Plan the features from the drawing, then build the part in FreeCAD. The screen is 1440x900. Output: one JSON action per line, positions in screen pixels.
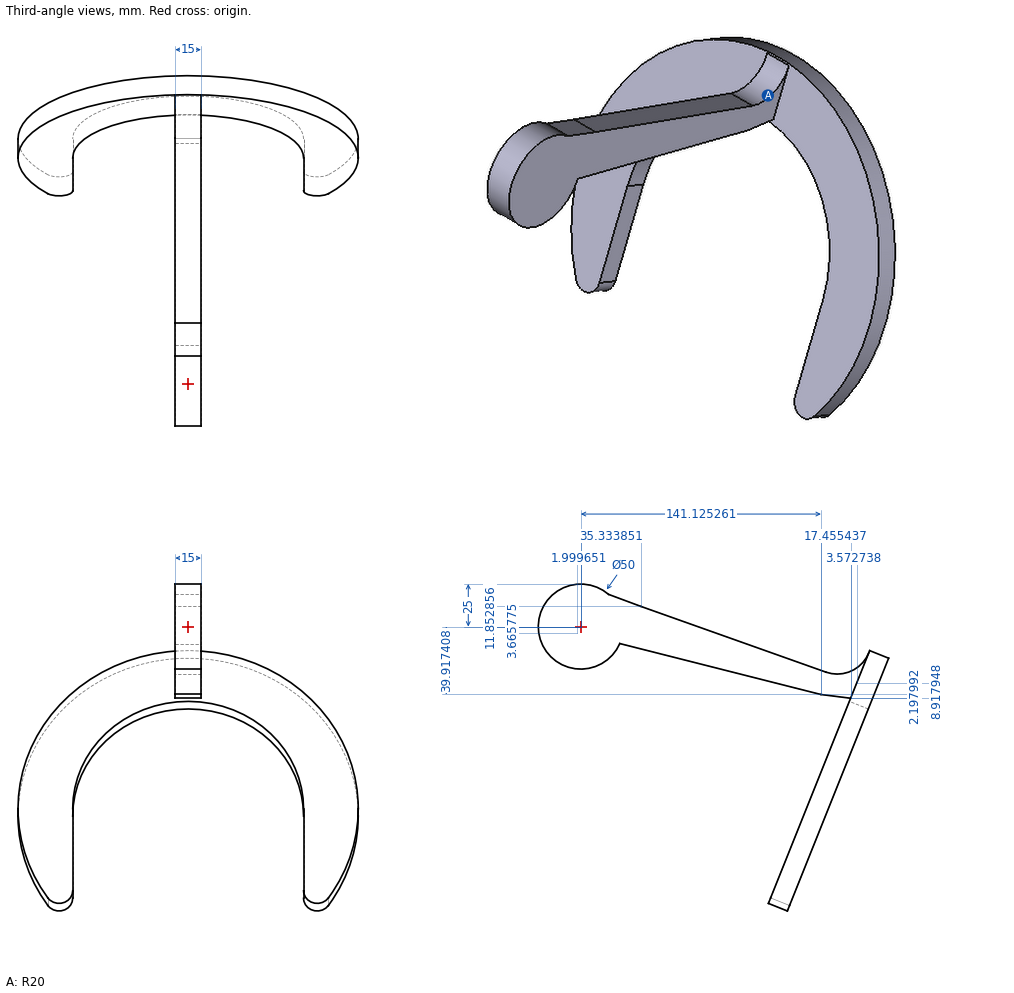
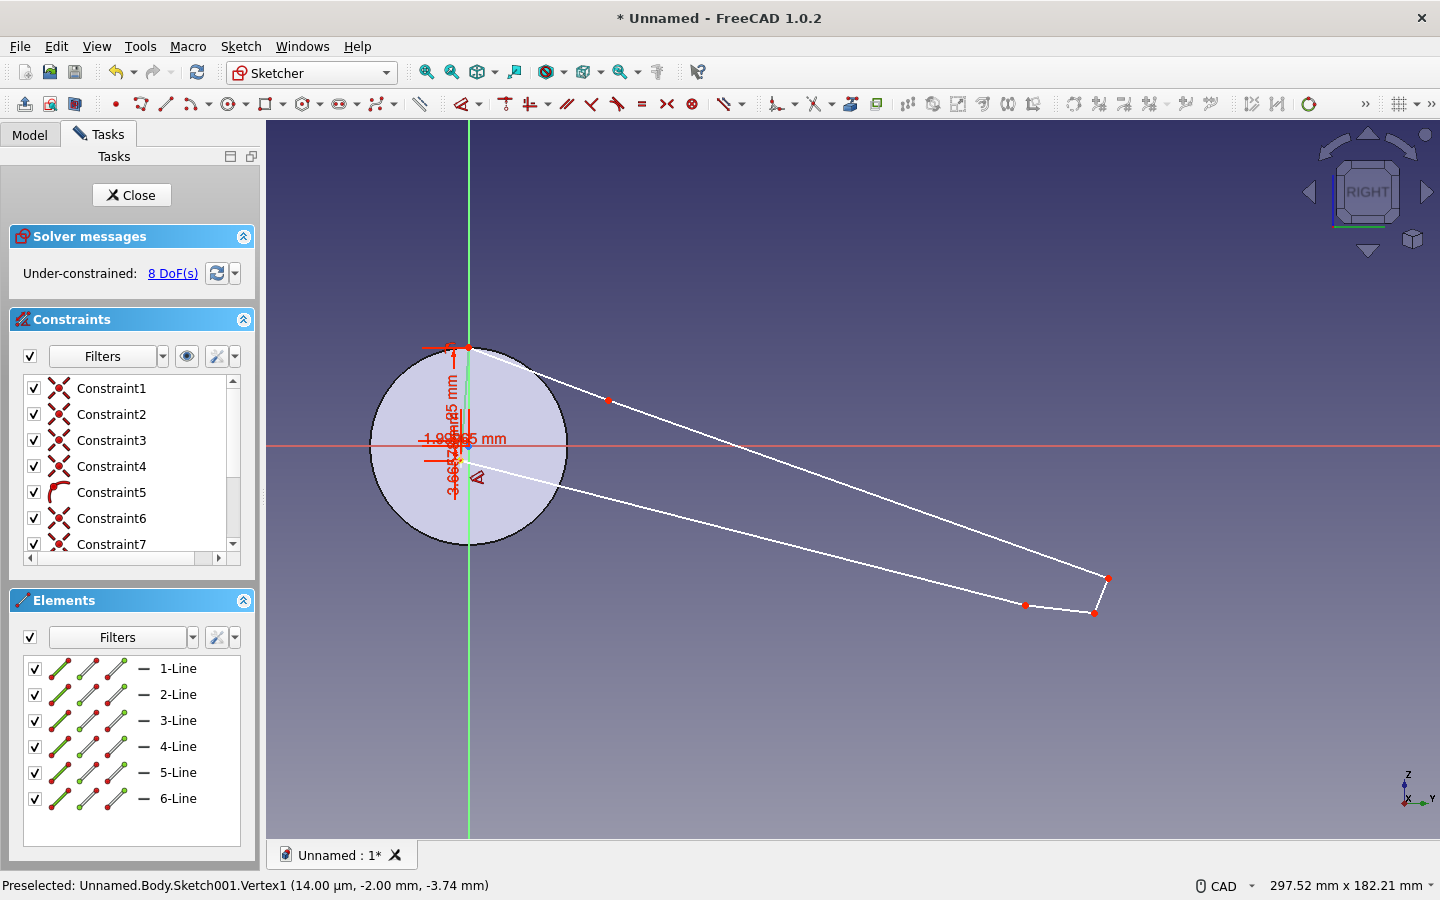
{"action": "scroll", "coordinate": [1046, 608], "scroll_direction": "up", "scroll_amount": 8}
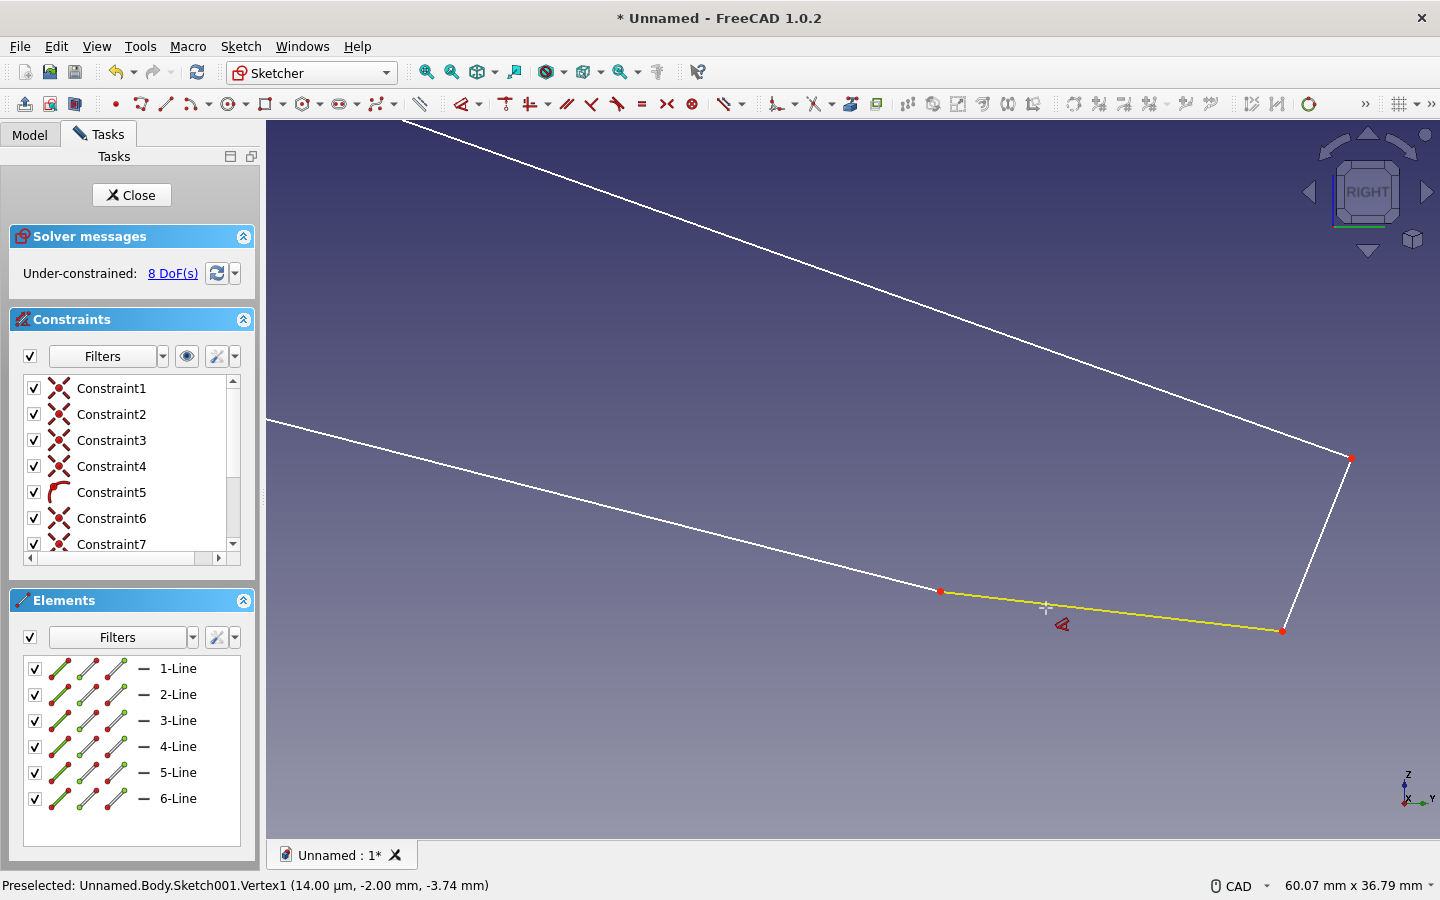
{"action": "left_click", "coordinate": [1043, 604]}
{"action": "left_click", "coordinate": [907, 612]}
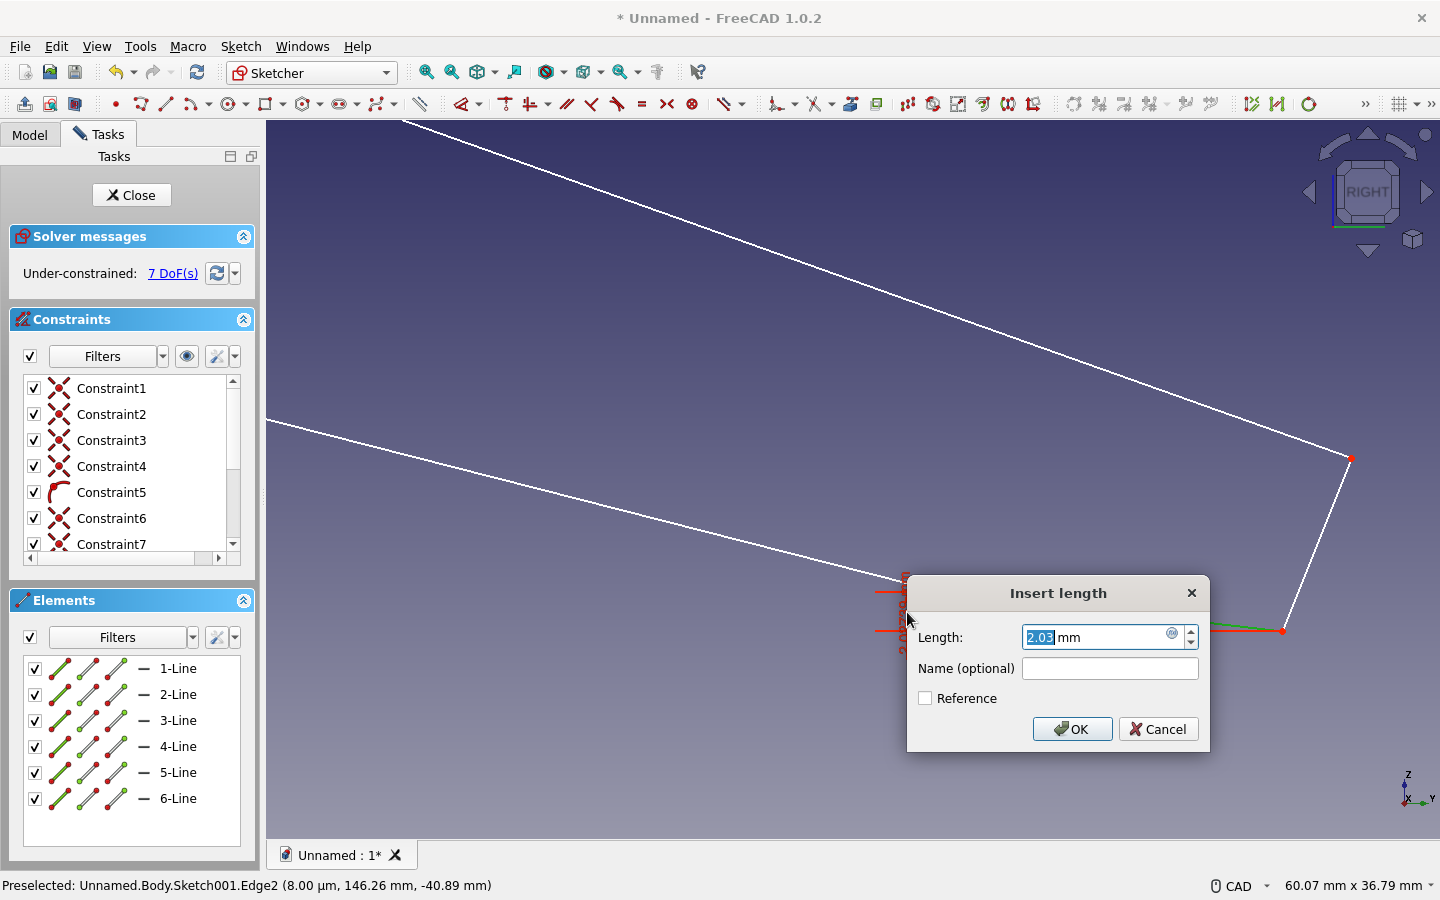
{"action": "type", "text": "2.197992"}
{"action": "key", "text": "Return"}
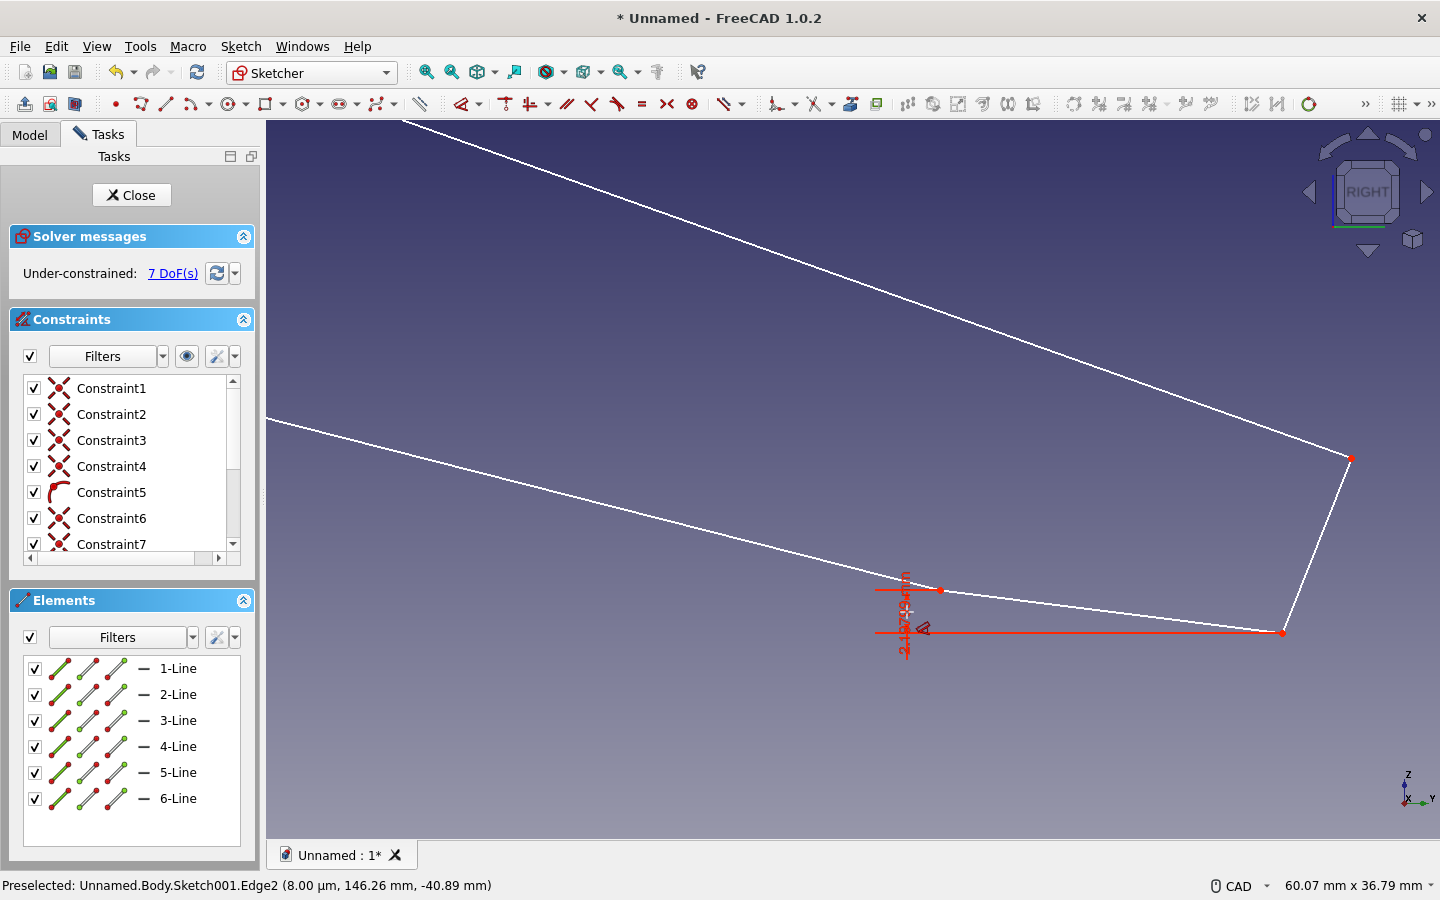
{"action": "scroll", "coordinate": [1046, 608], "scroll_direction": "down", "scroll_amount": 8}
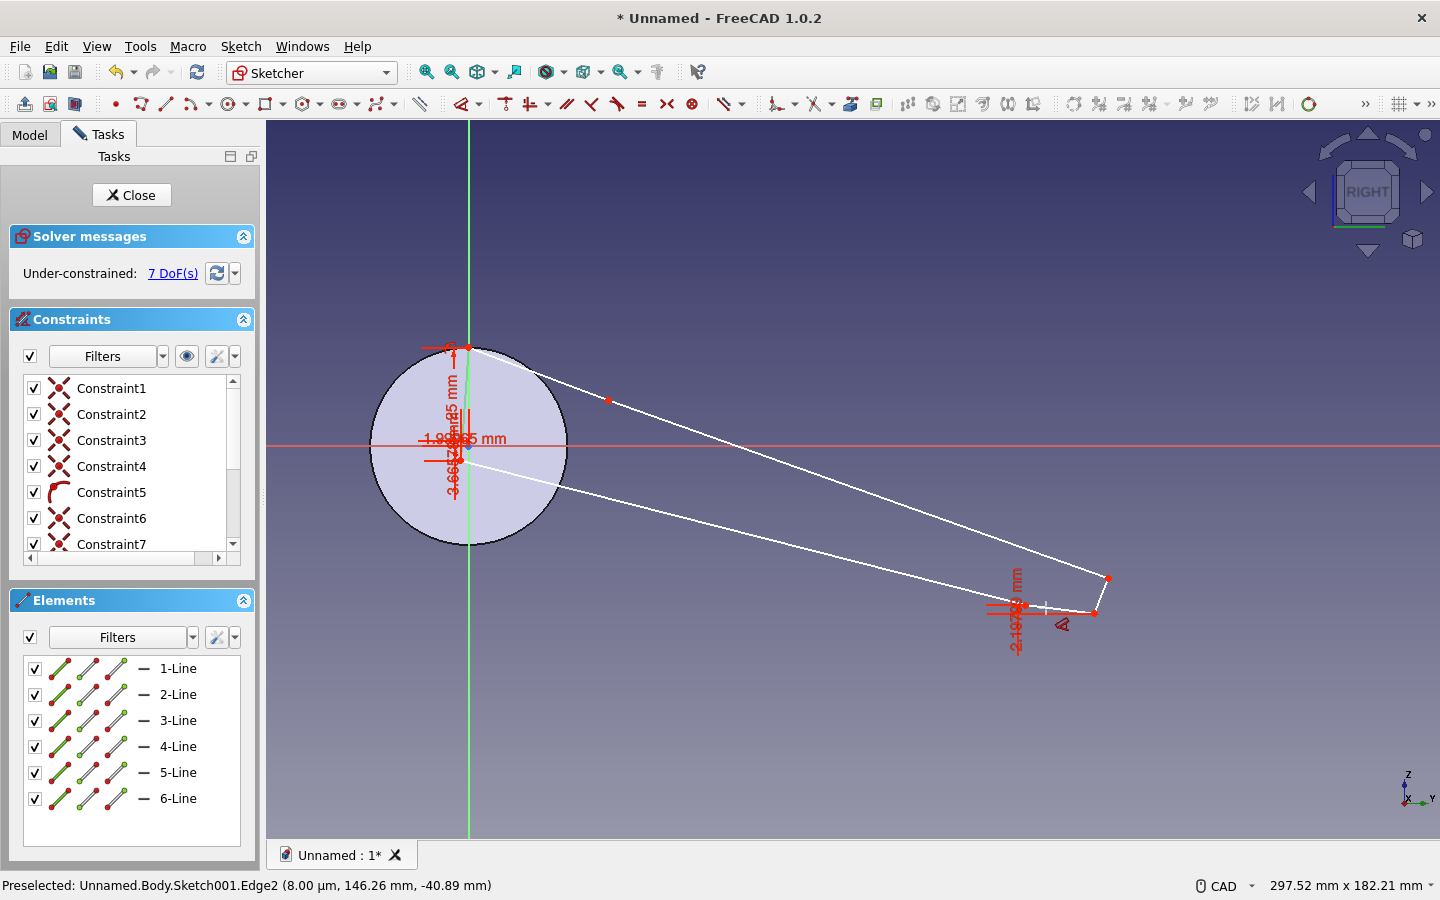
{"action": "scroll", "coordinate": [1098, 603], "scroll_direction": "up", "scroll_amount": 6}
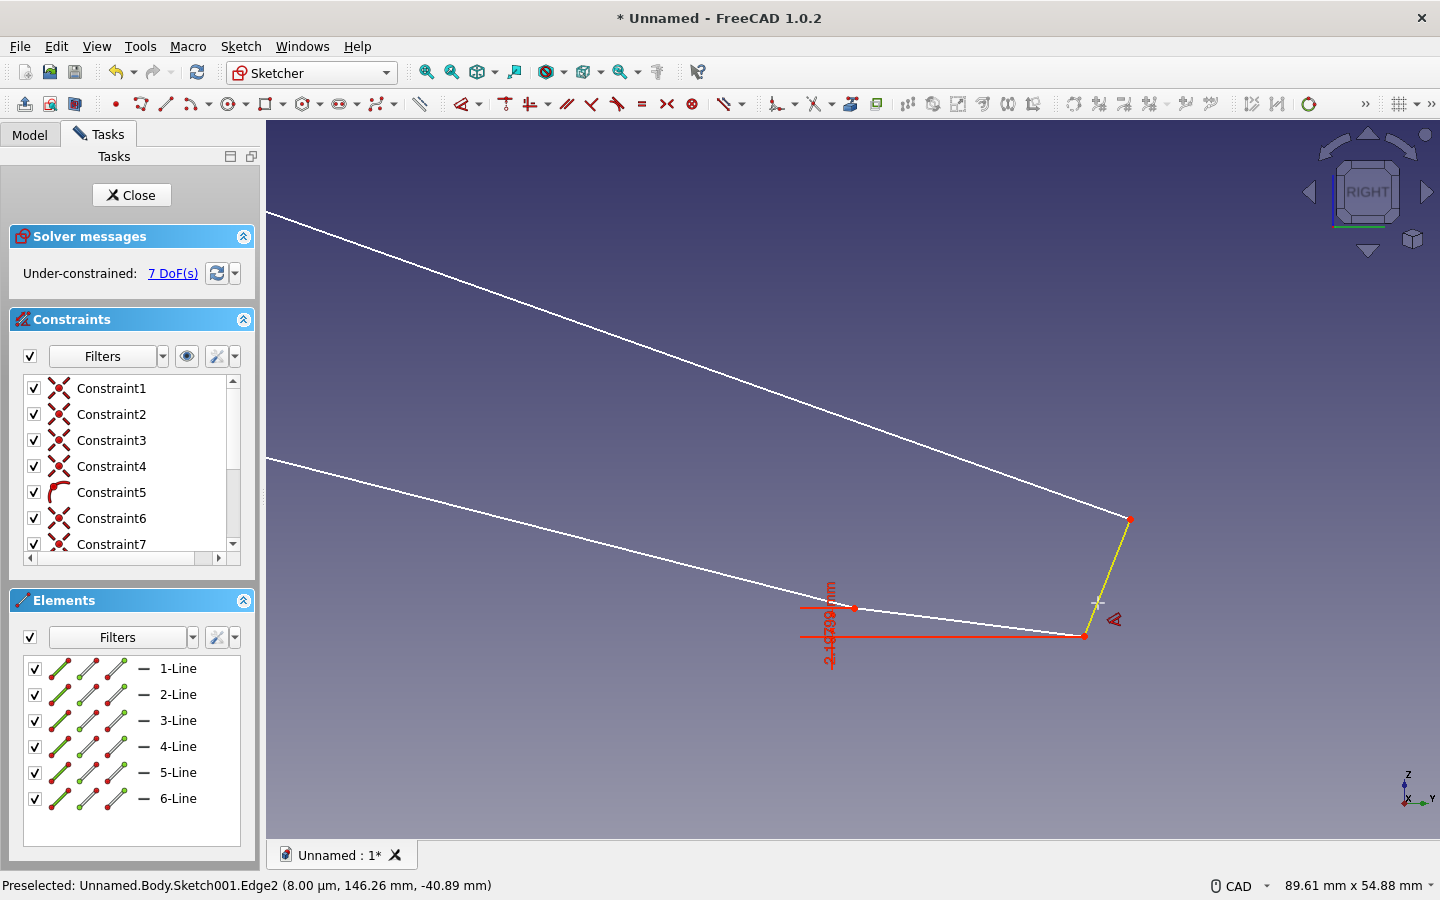
{"action": "left_click", "coordinate": [1098, 602]}
{"action": "left_click", "coordinate": [1107, 671]}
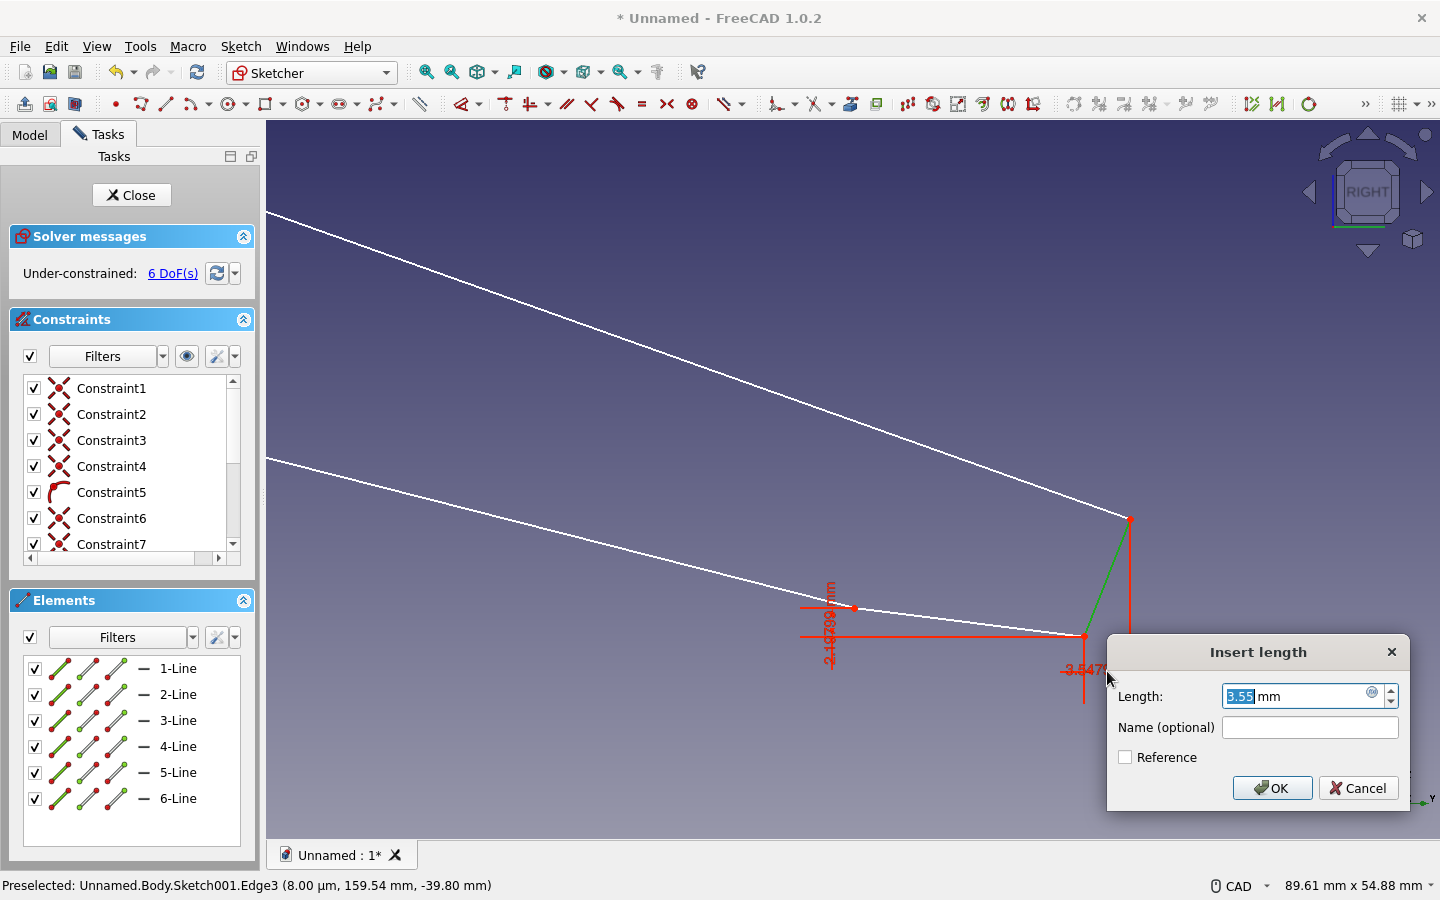
{"action": "type", "text": "3.572738"}
{"action": "key", "text": "Return"}